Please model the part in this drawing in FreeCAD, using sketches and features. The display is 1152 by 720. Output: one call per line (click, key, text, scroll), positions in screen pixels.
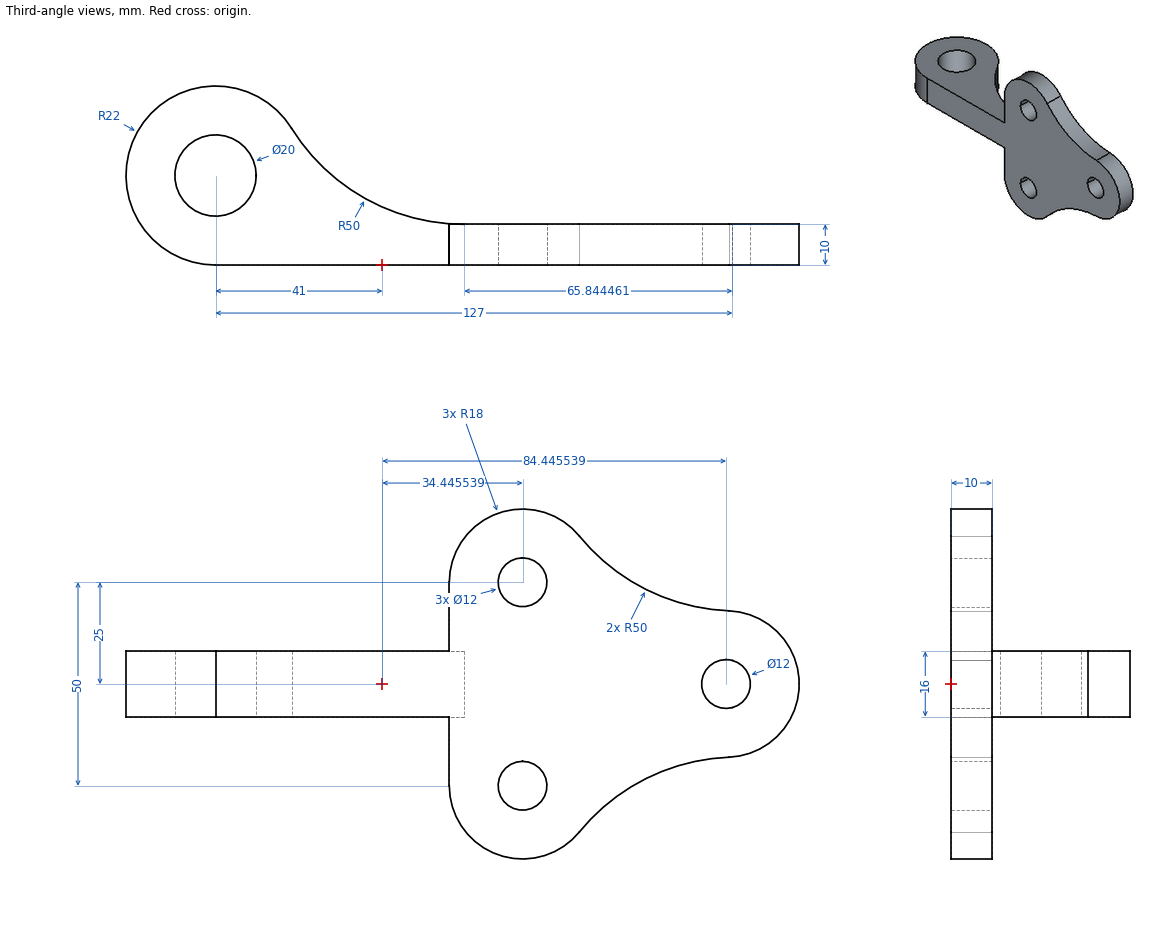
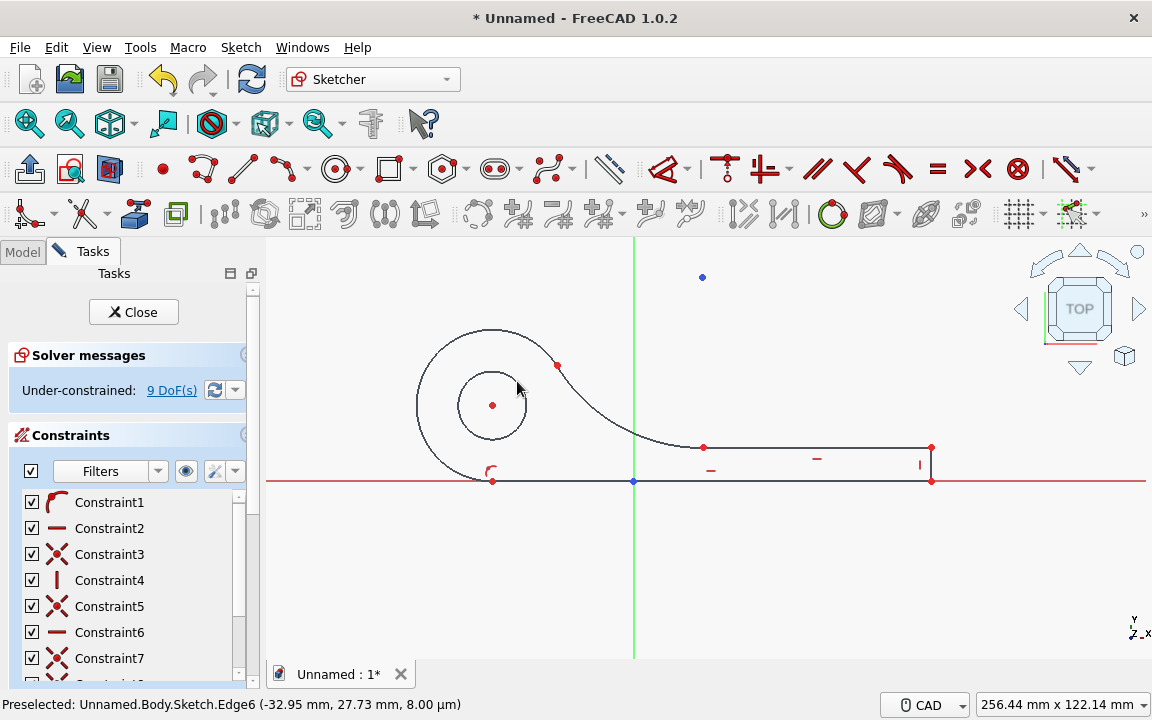
scroll(624, 481, up, 2)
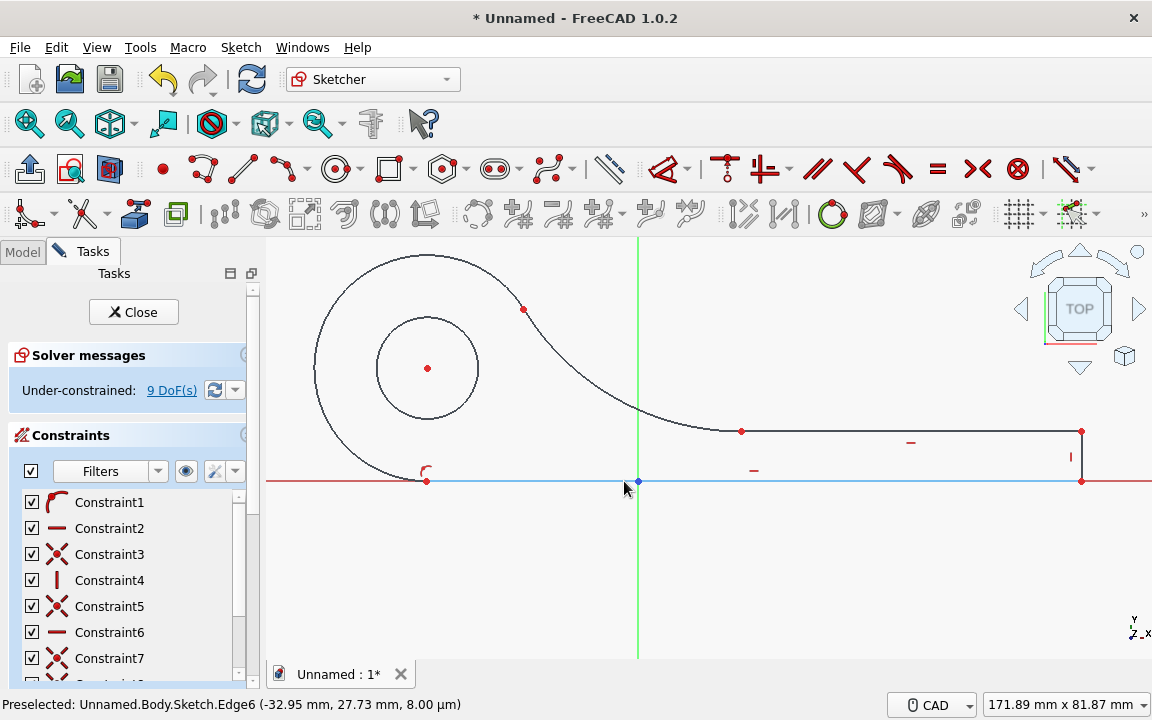
click(623, 481)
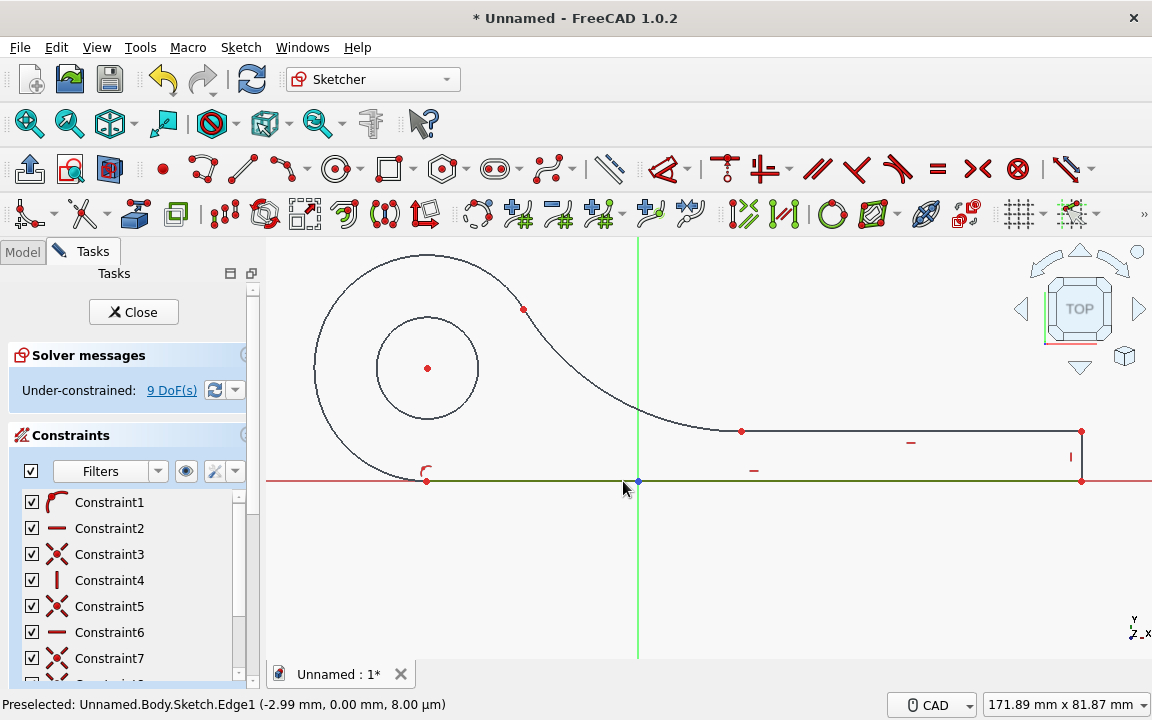
click(320, 404)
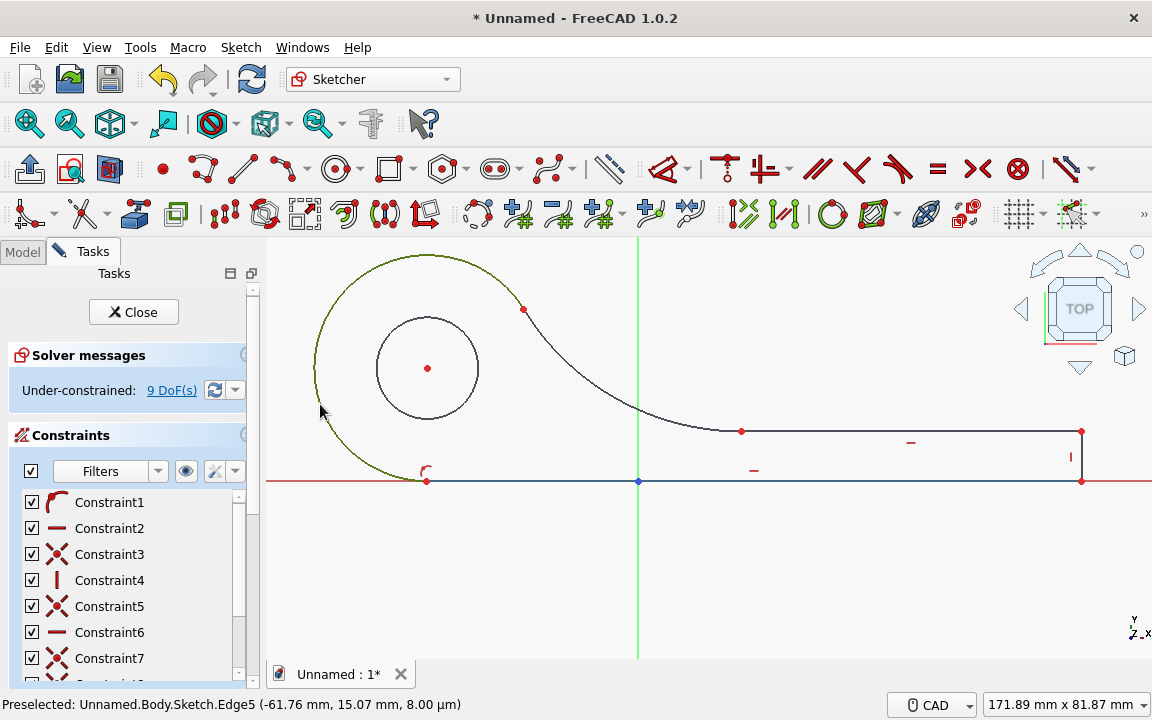
key(t)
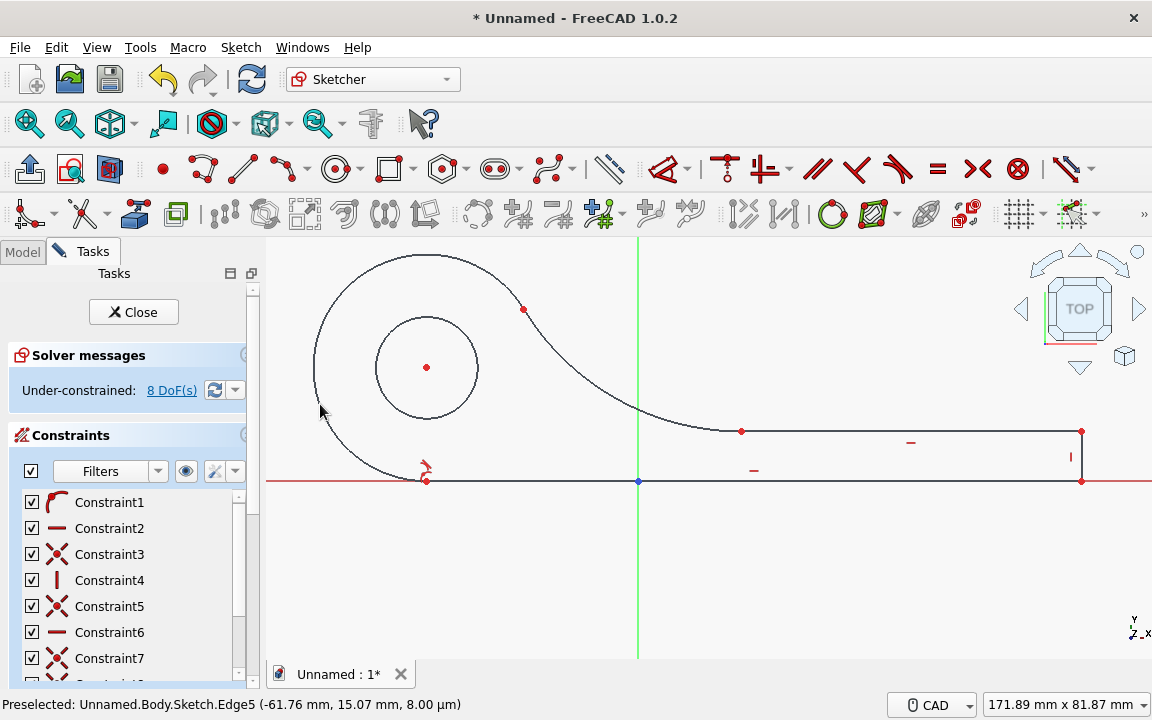
click(574, 369)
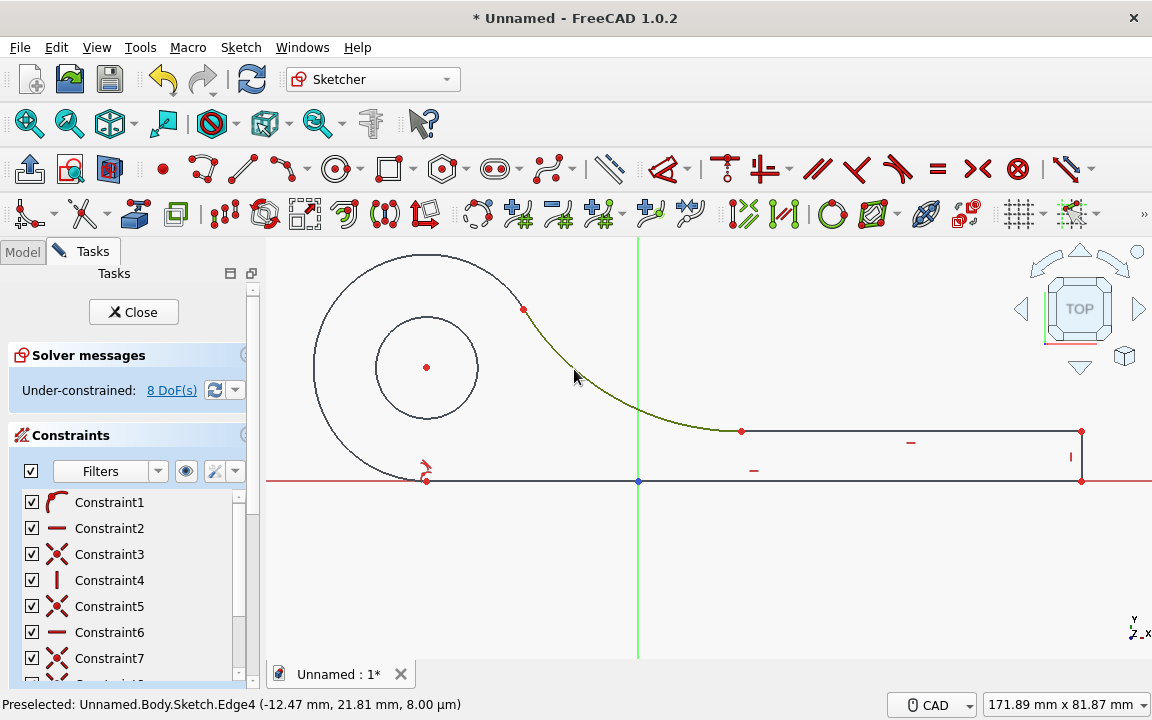
click(319, 404)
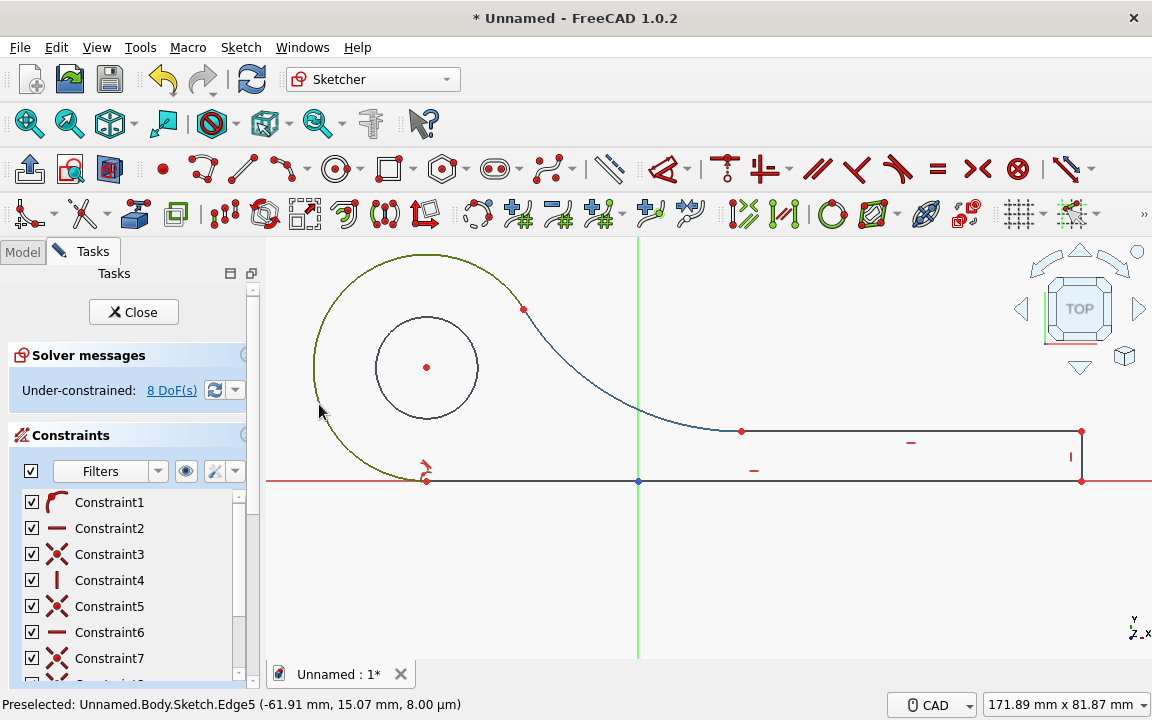
key(t)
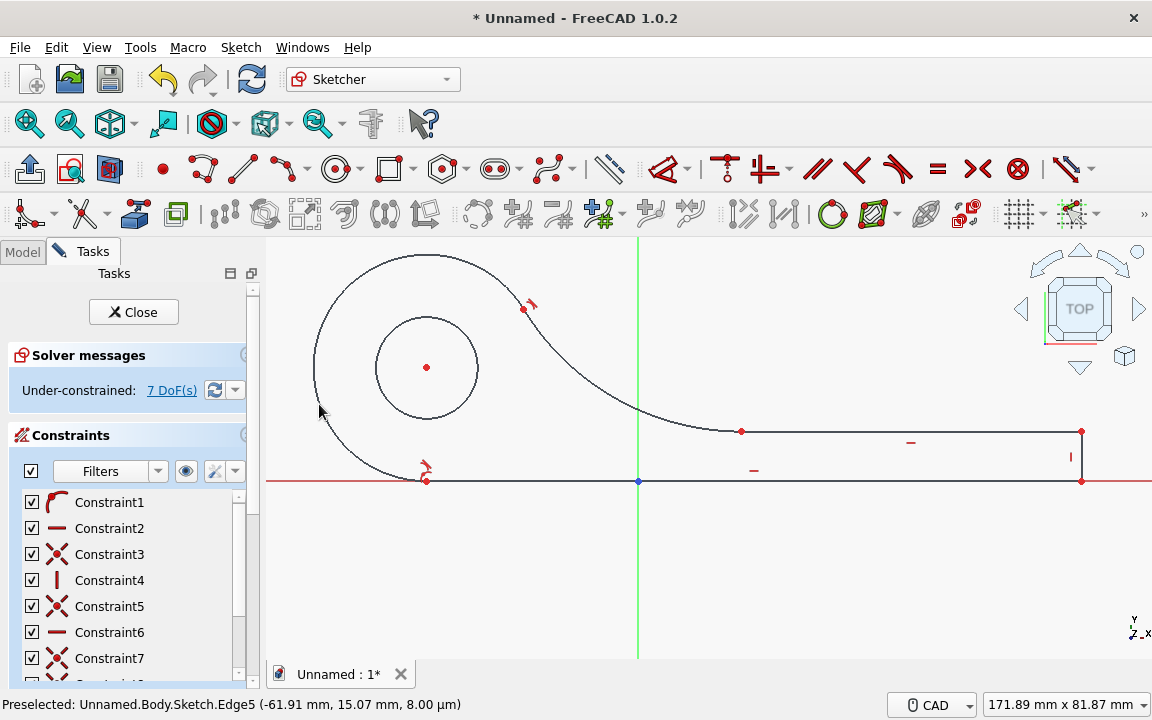
key(d)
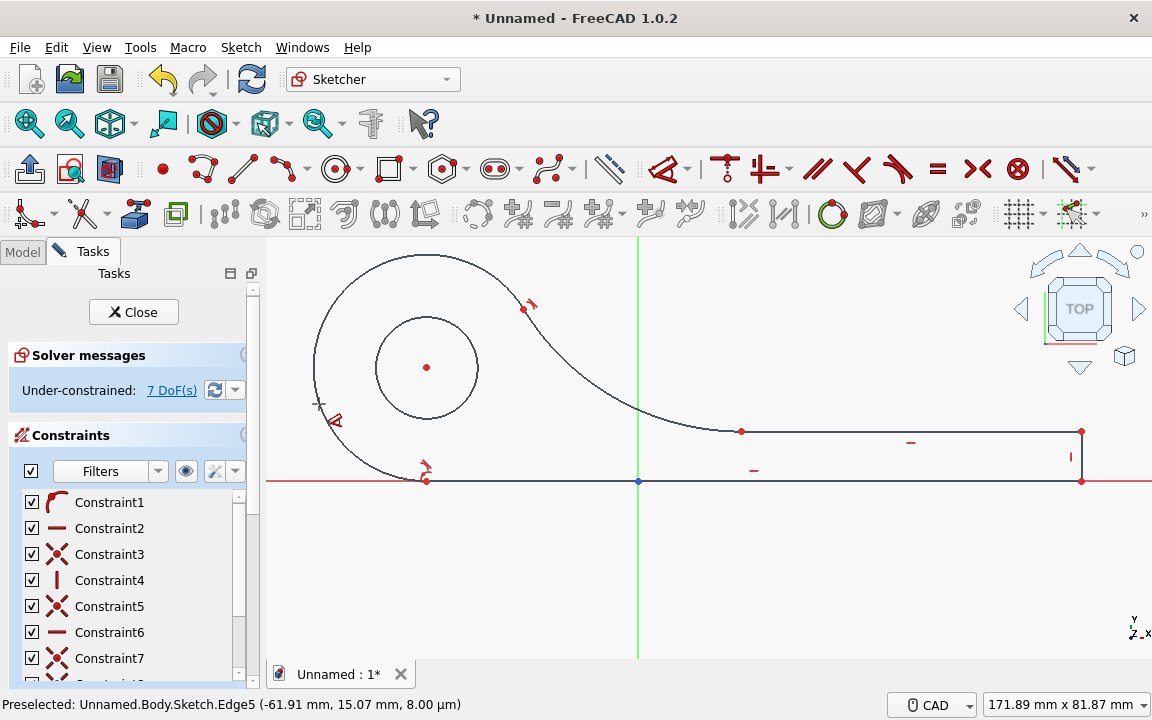
click(574, 369)
click(553, 393)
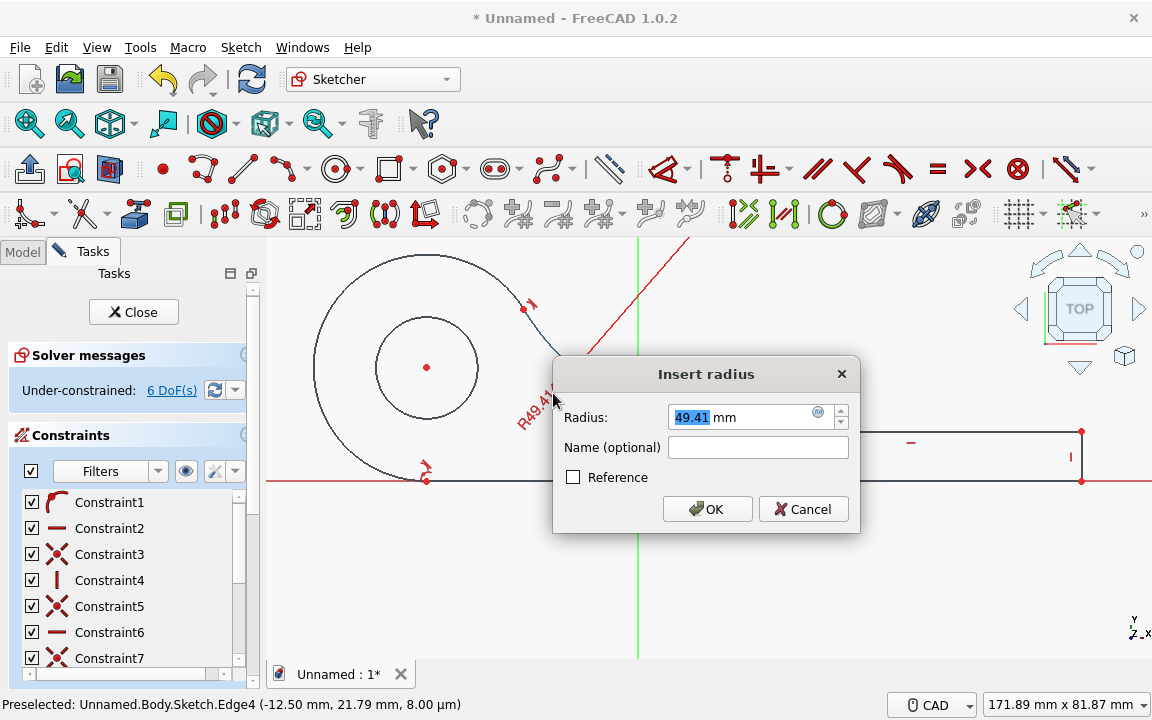
text(50)
key(Return)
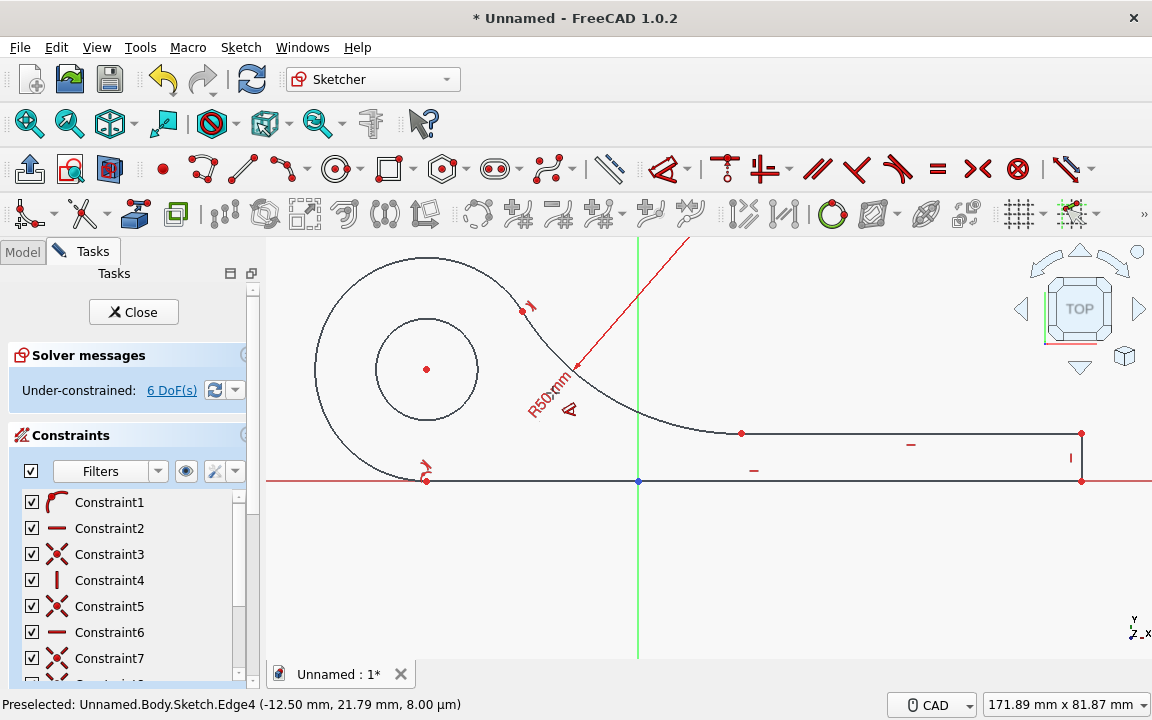
click(321, 405)
click(315, 280)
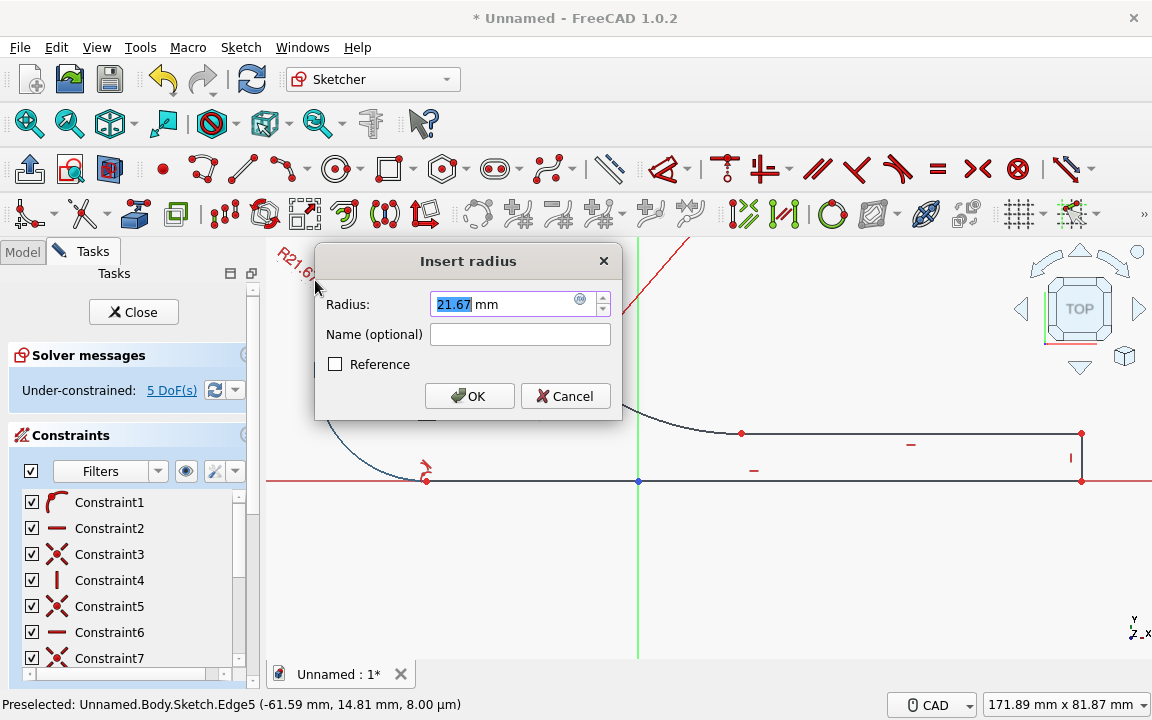
text(22)
key(Return)